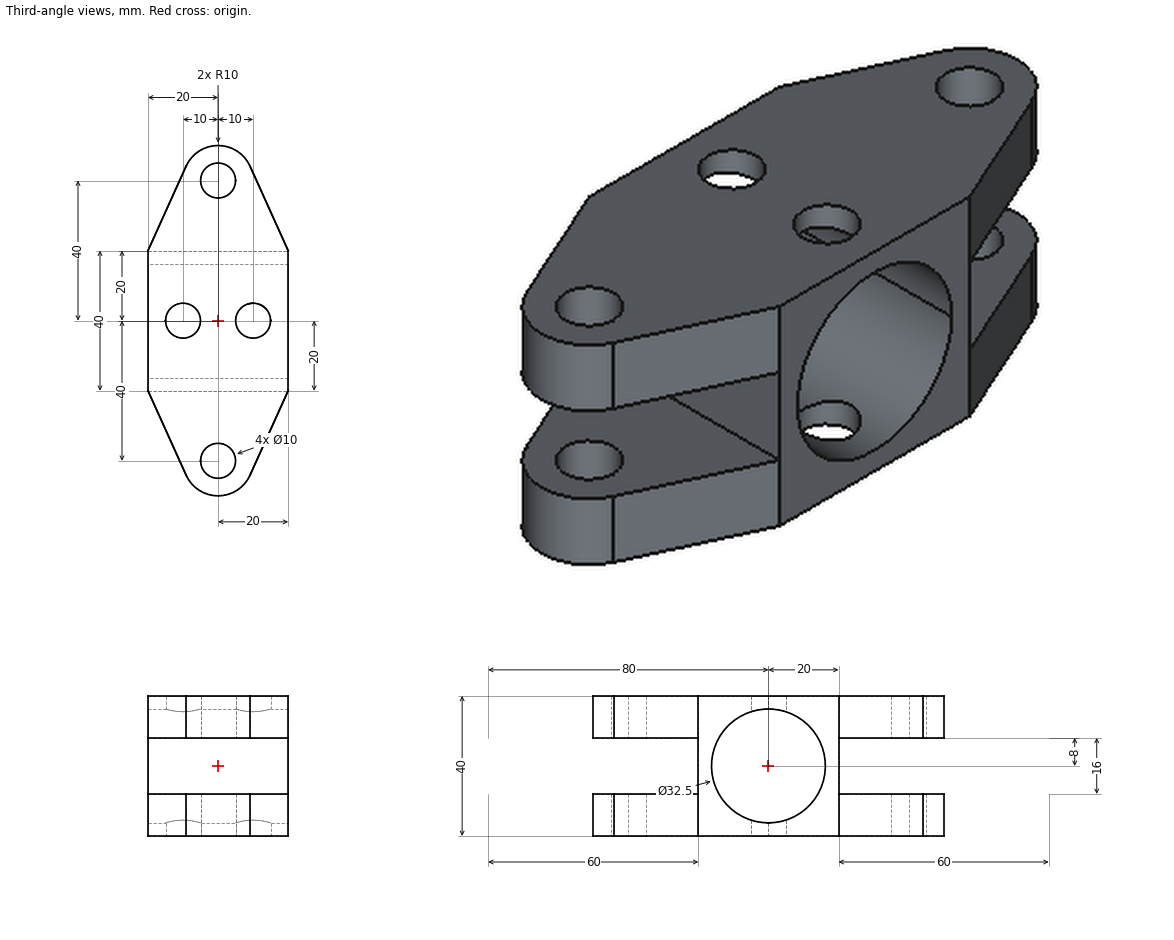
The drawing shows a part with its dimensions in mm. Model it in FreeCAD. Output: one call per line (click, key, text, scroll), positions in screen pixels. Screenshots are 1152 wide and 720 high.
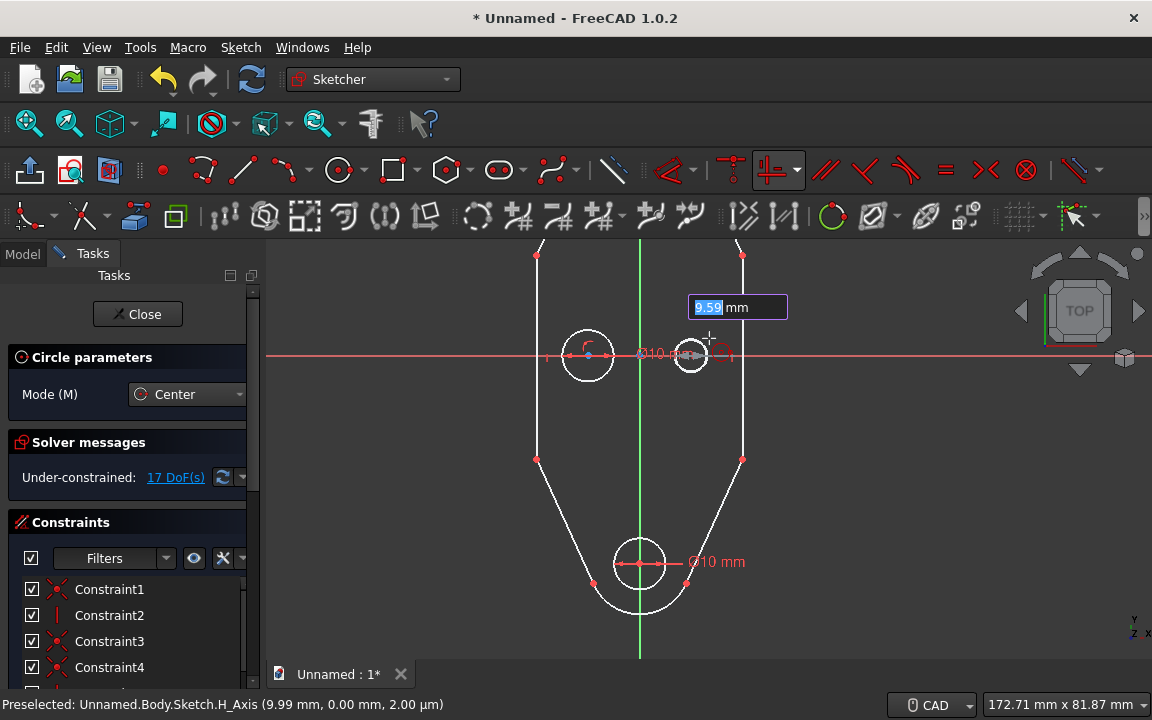
text(10)
key(Return)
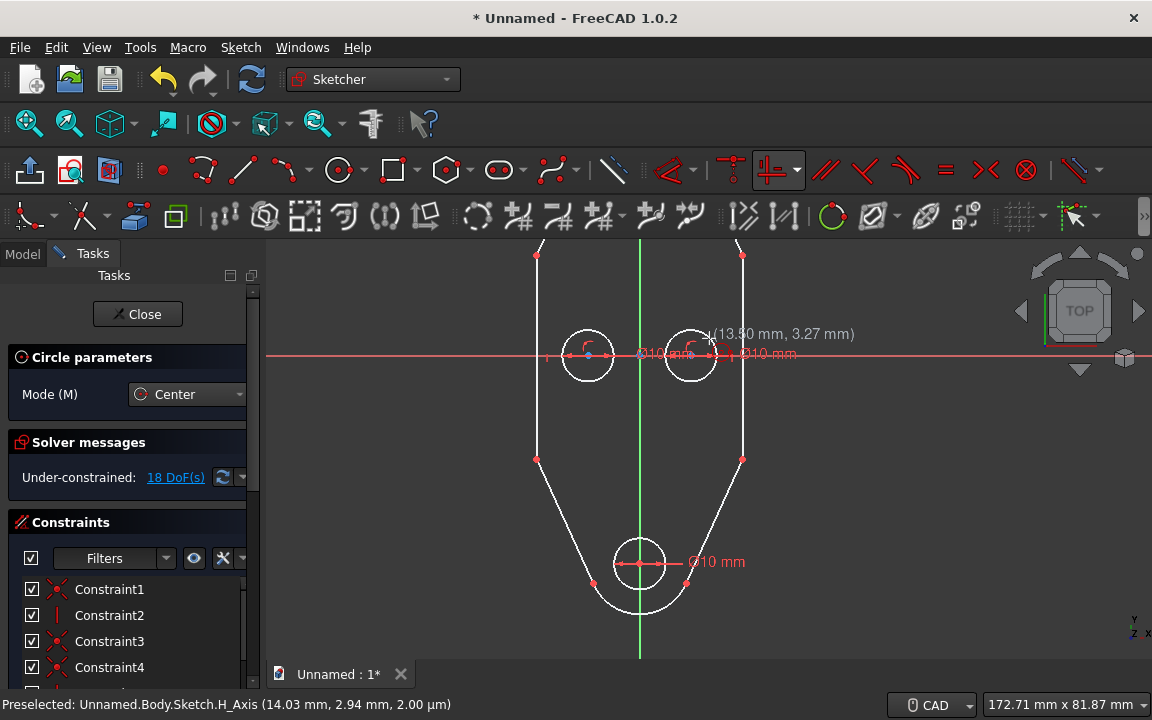
scroll(641, 562, down, 3)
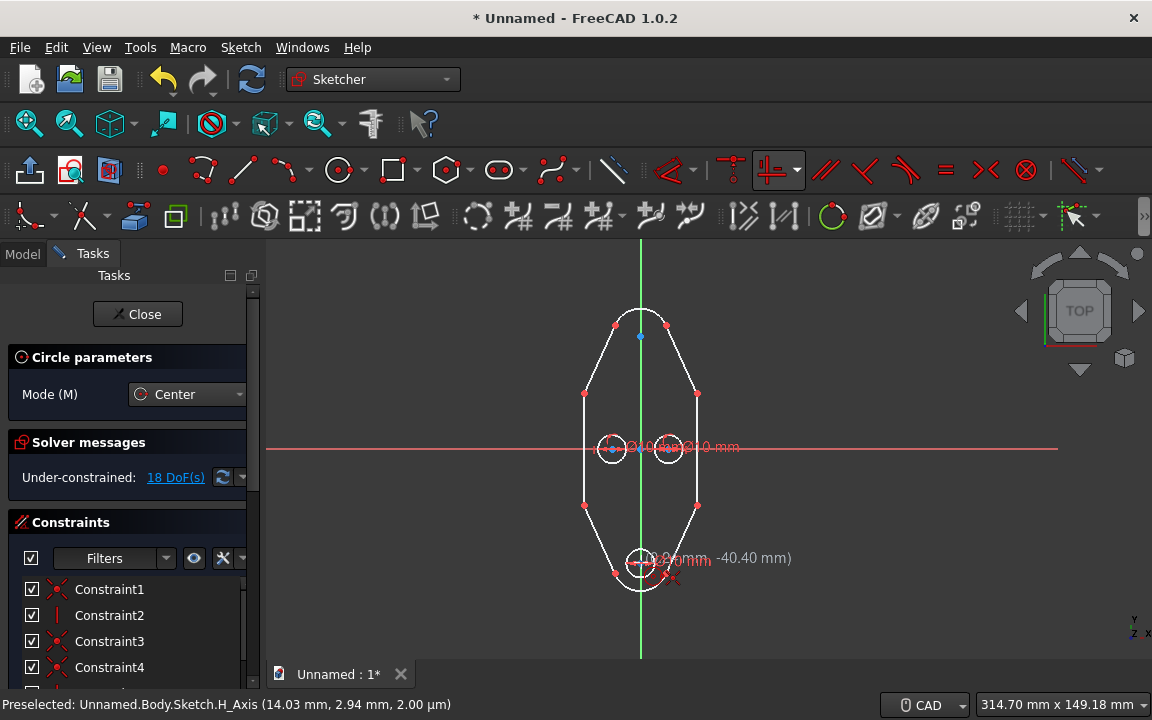
scroll(641, 337, up, 3)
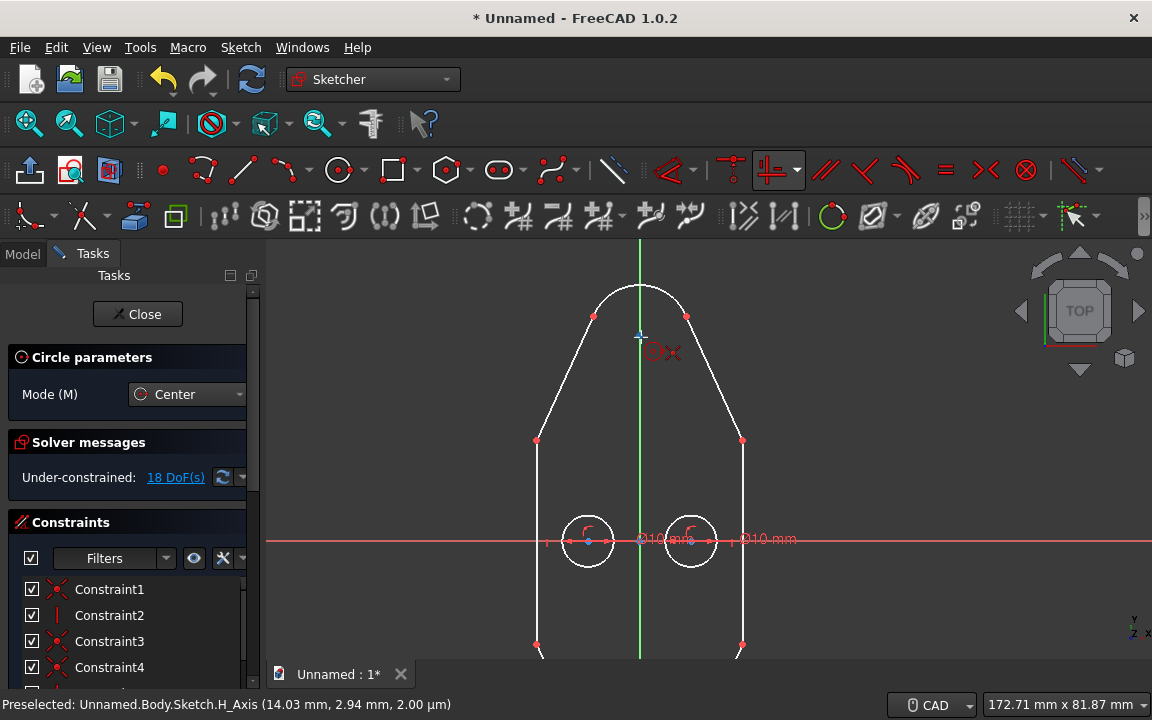
click(640, 336)
move(658, 318)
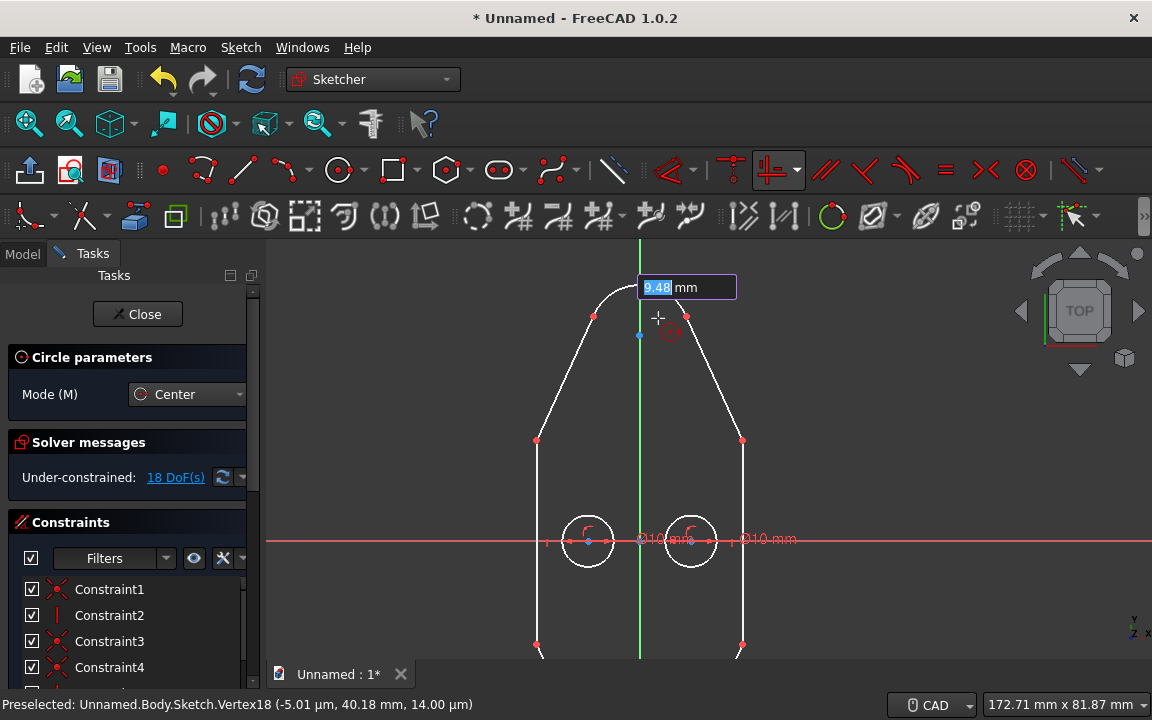
text(10)
key(Return)
key(Escape)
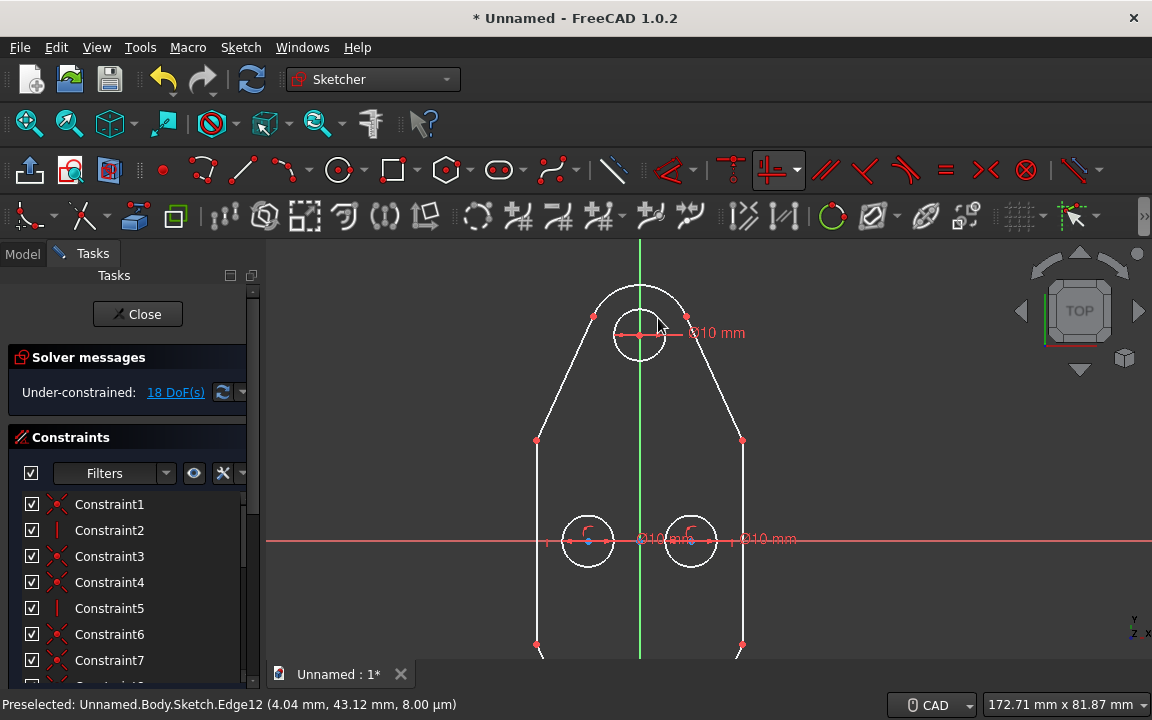
click(576, 354)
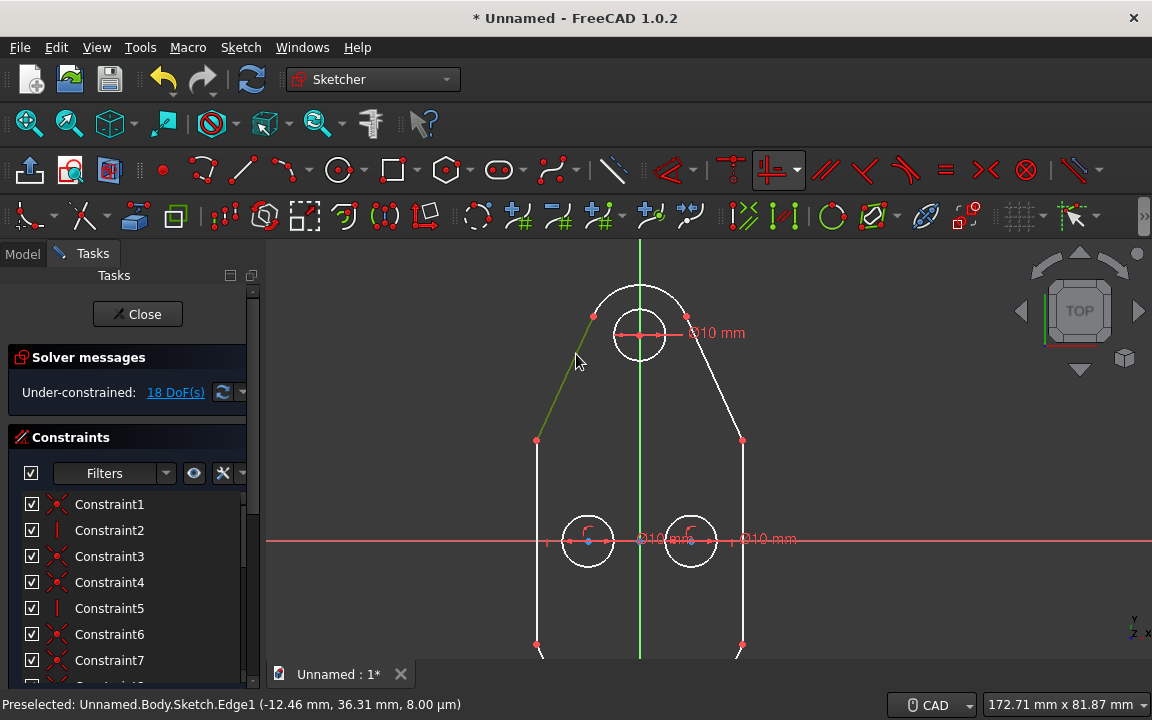
click(663, 291)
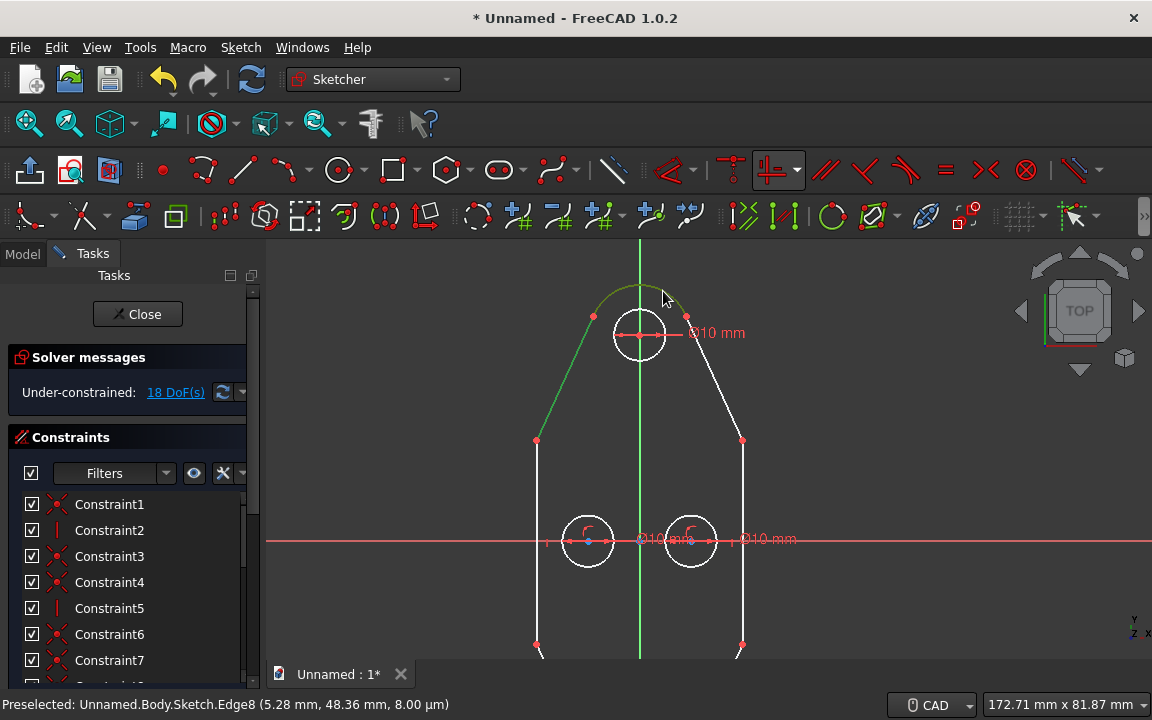
click(906, 170)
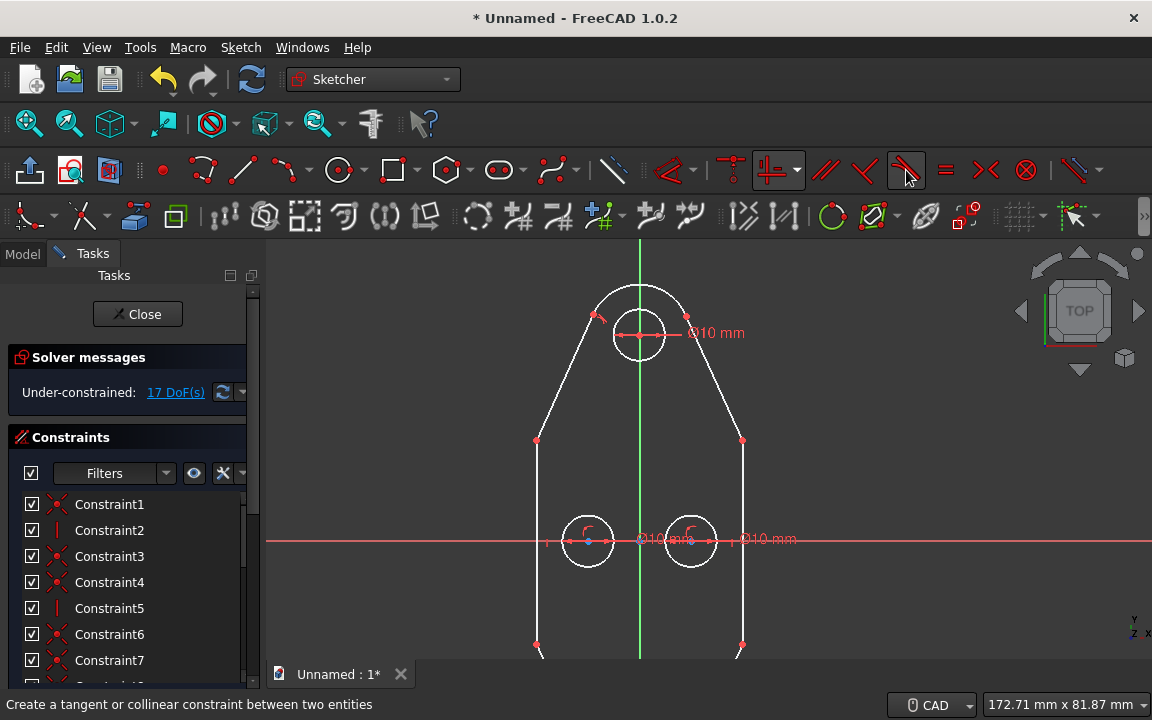
scroll(641, 337, down, 3)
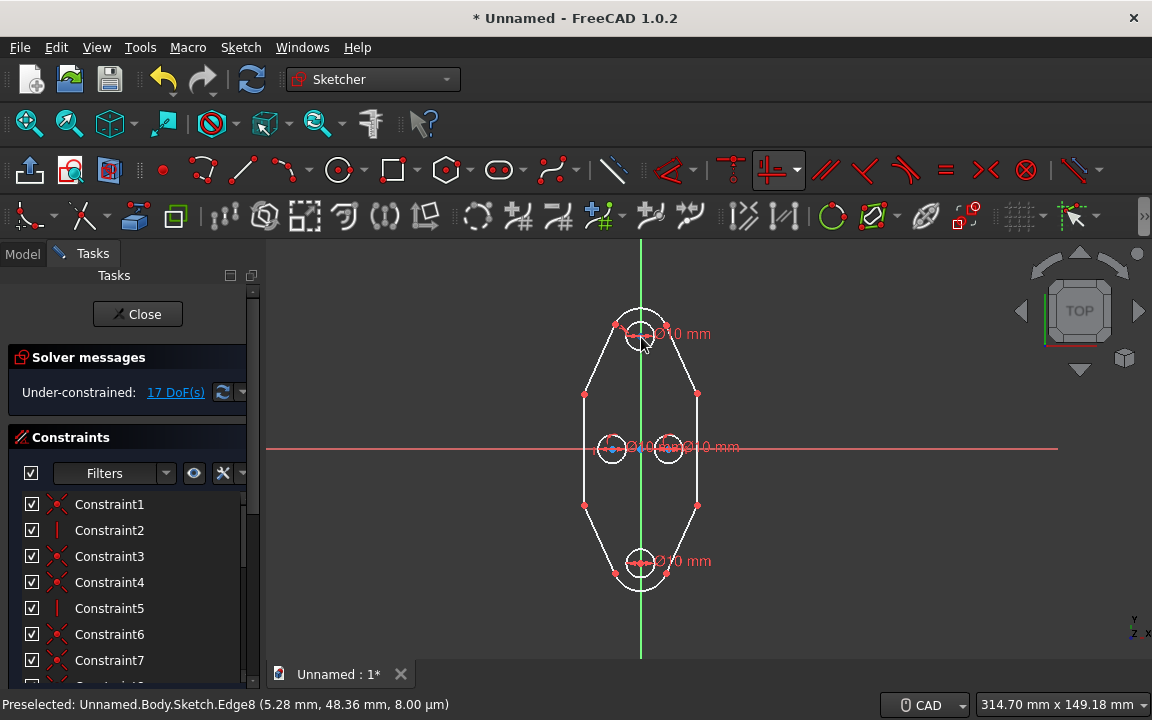
click(593, 526)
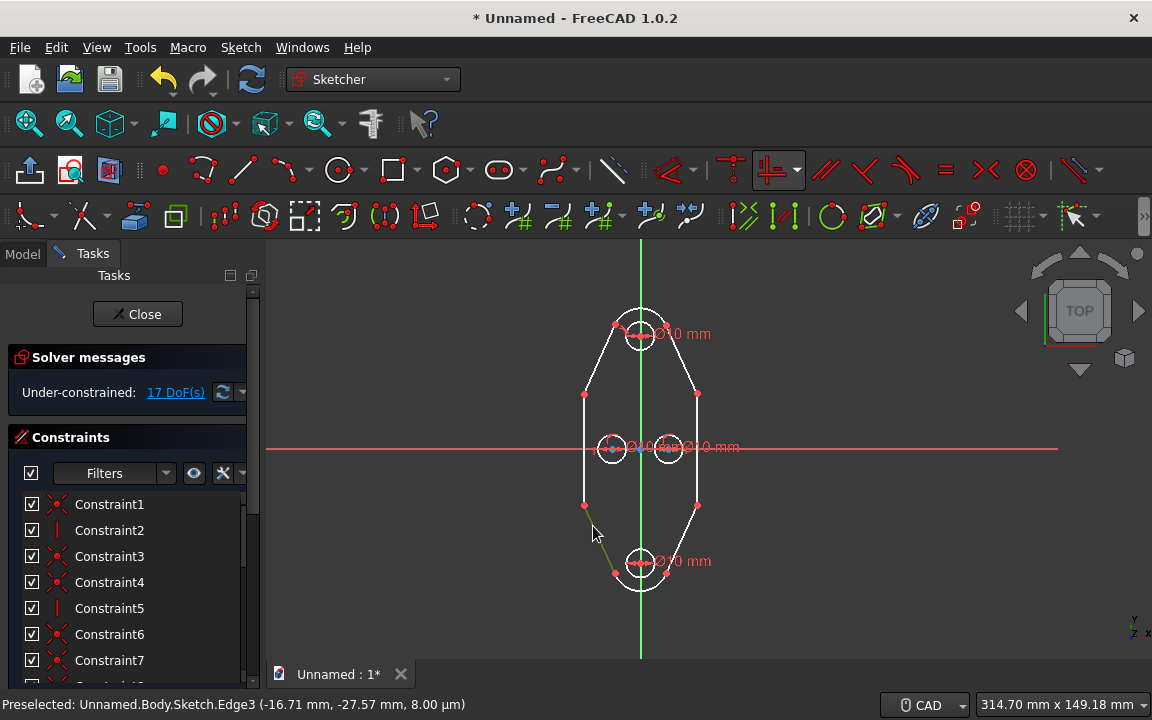
click(628, 588)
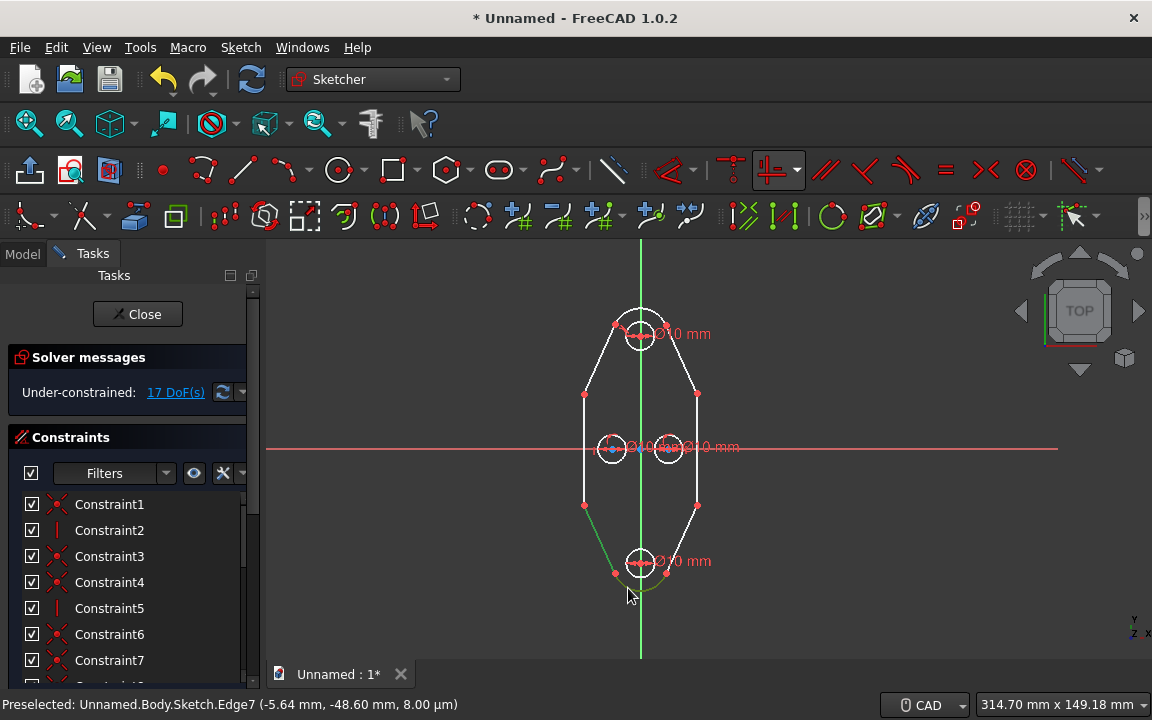
click(906, 170)